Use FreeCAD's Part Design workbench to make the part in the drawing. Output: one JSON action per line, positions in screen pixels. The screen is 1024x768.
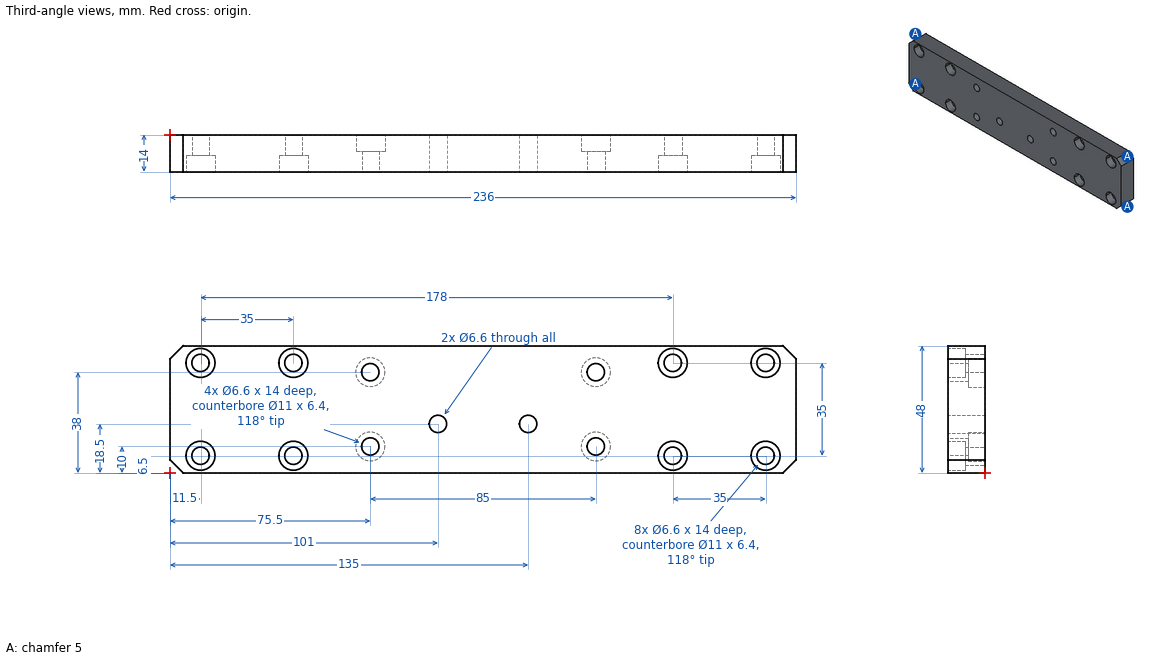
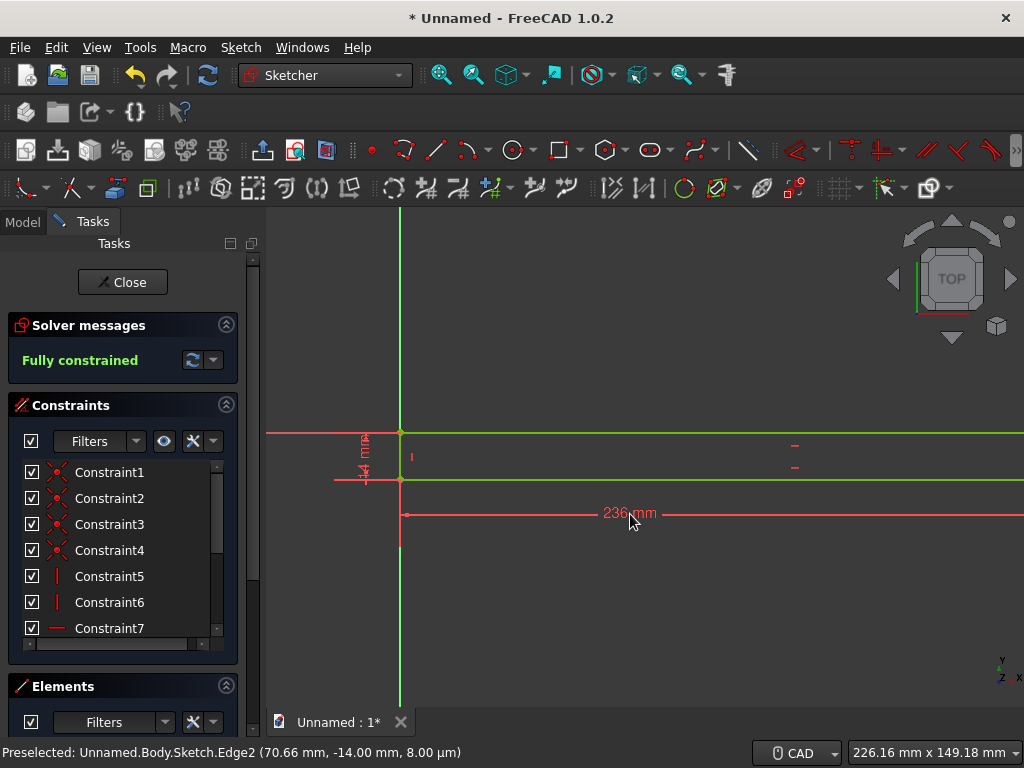
{"action": "left_click", "coordinate": [123, 282]}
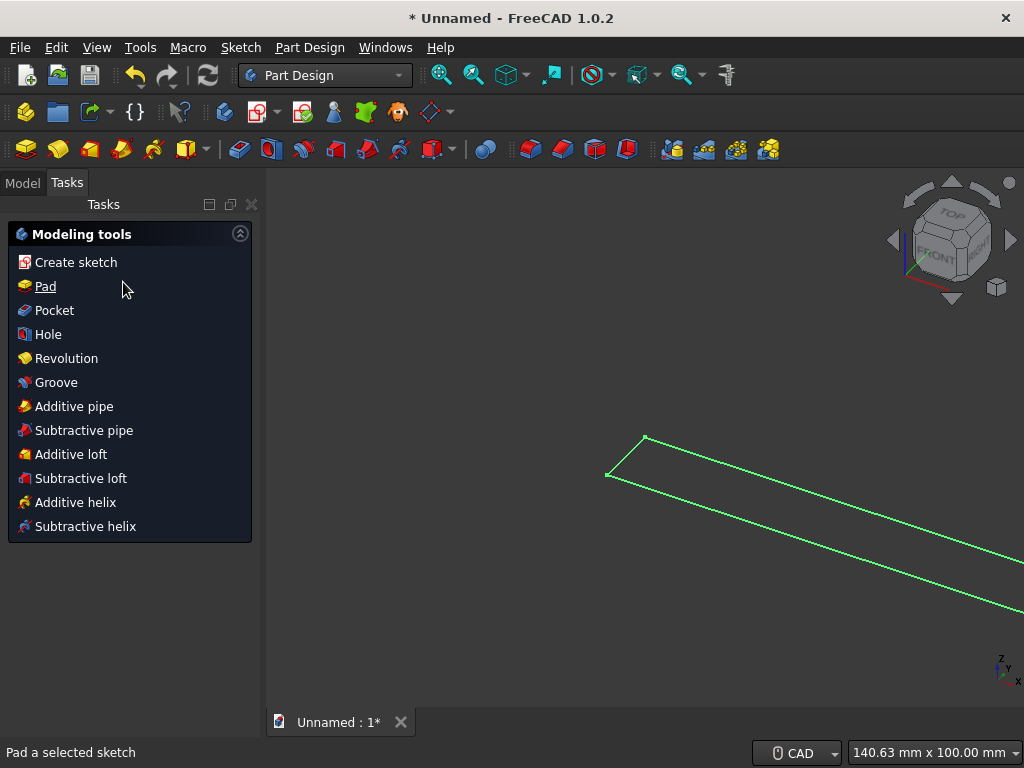
{"action": "left_click", "coordinate": [26, 150]}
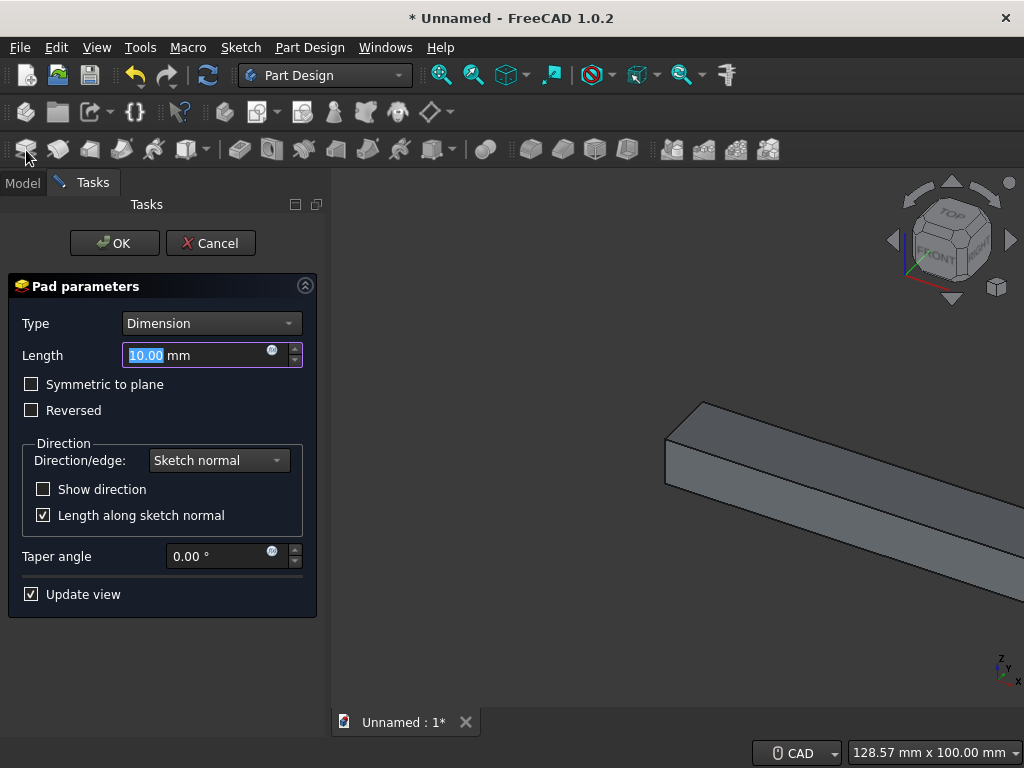
{"action": "type", "text": "48"}
{"action": "key", "text": "Tab"}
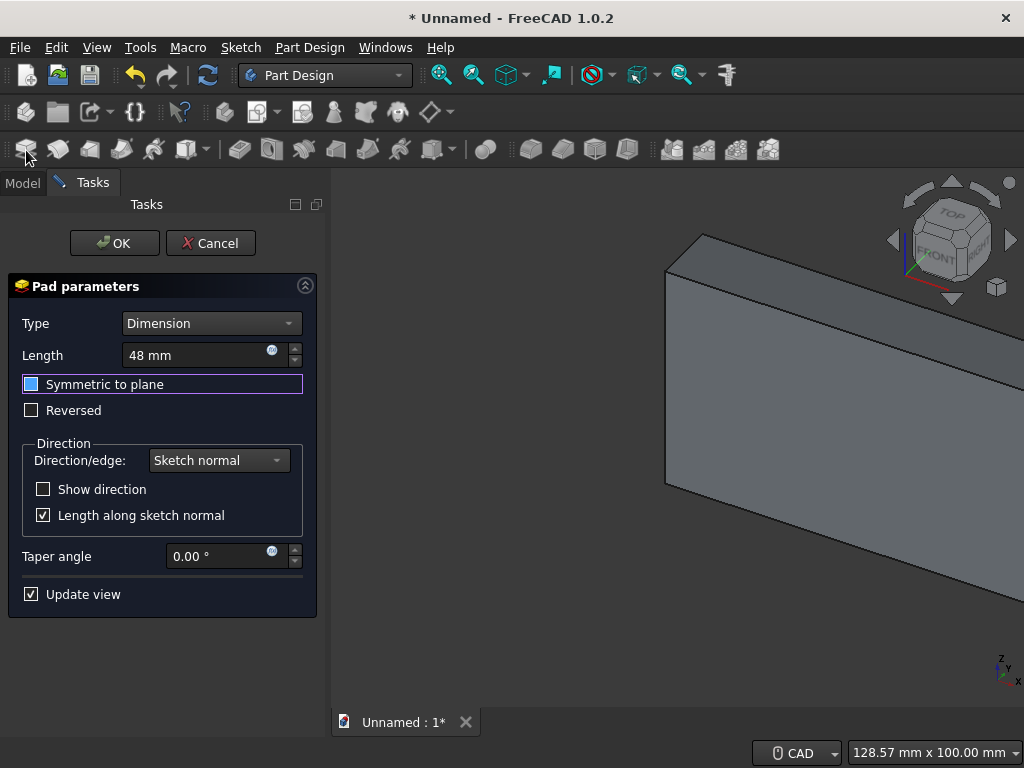
{"action": "left_click", "coordinate": [115, 243]}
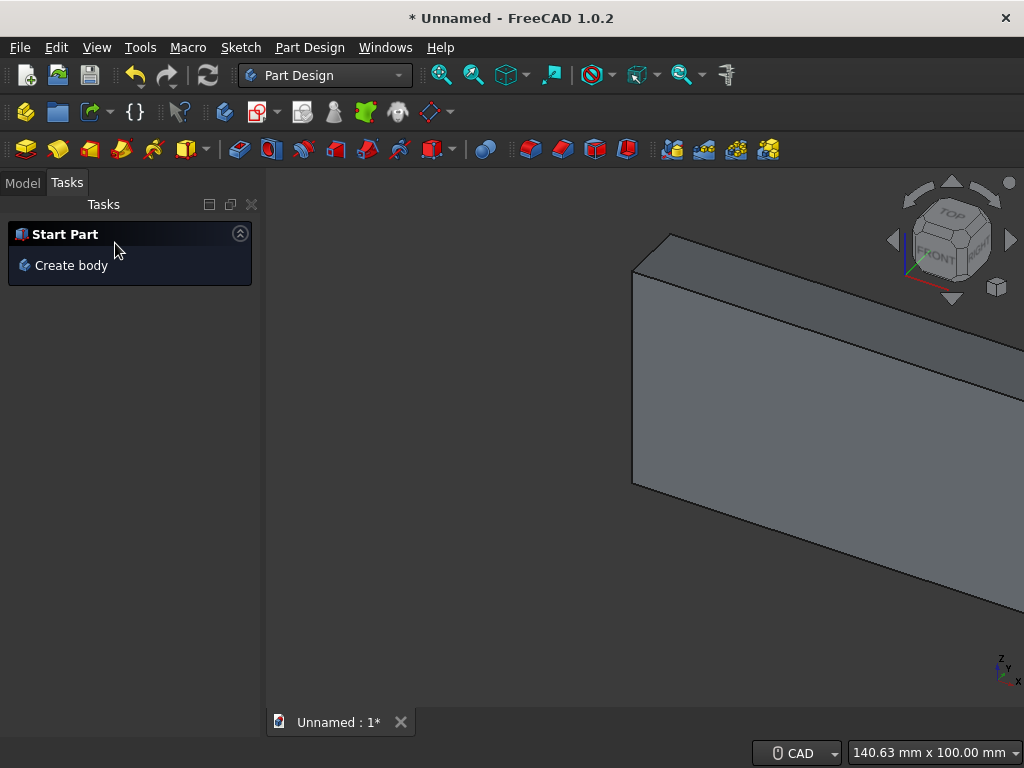
{"action": "left_click", "coordinate": [442, 76]}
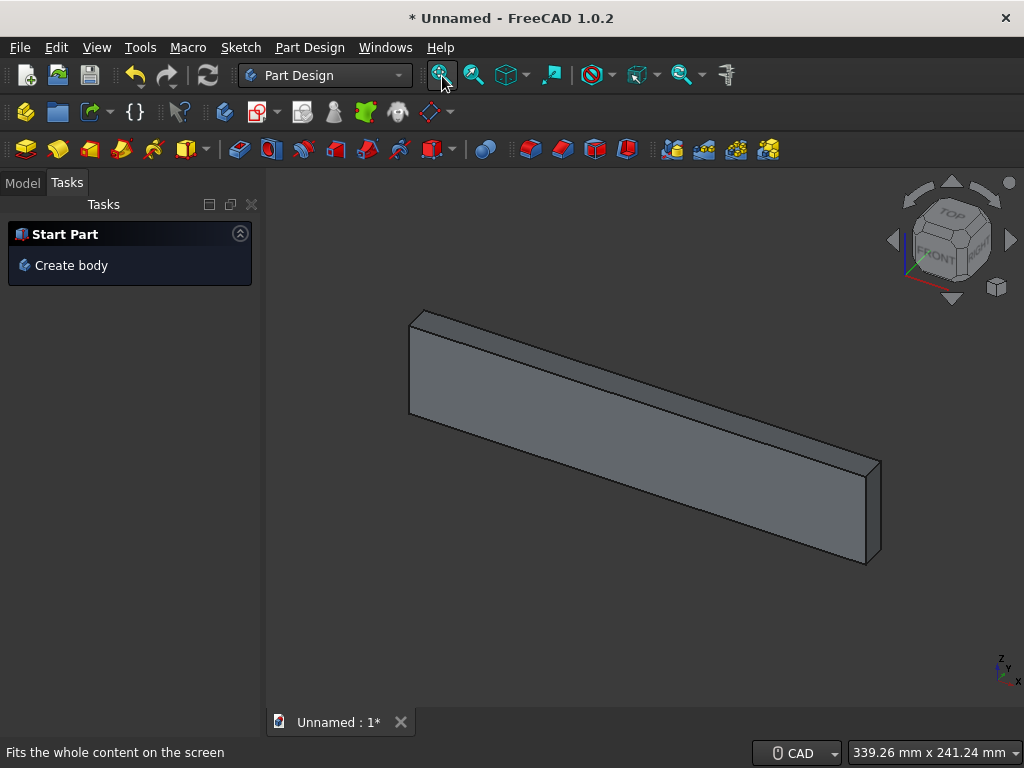
{"action": "left_click", "coordinate": [768, 487]}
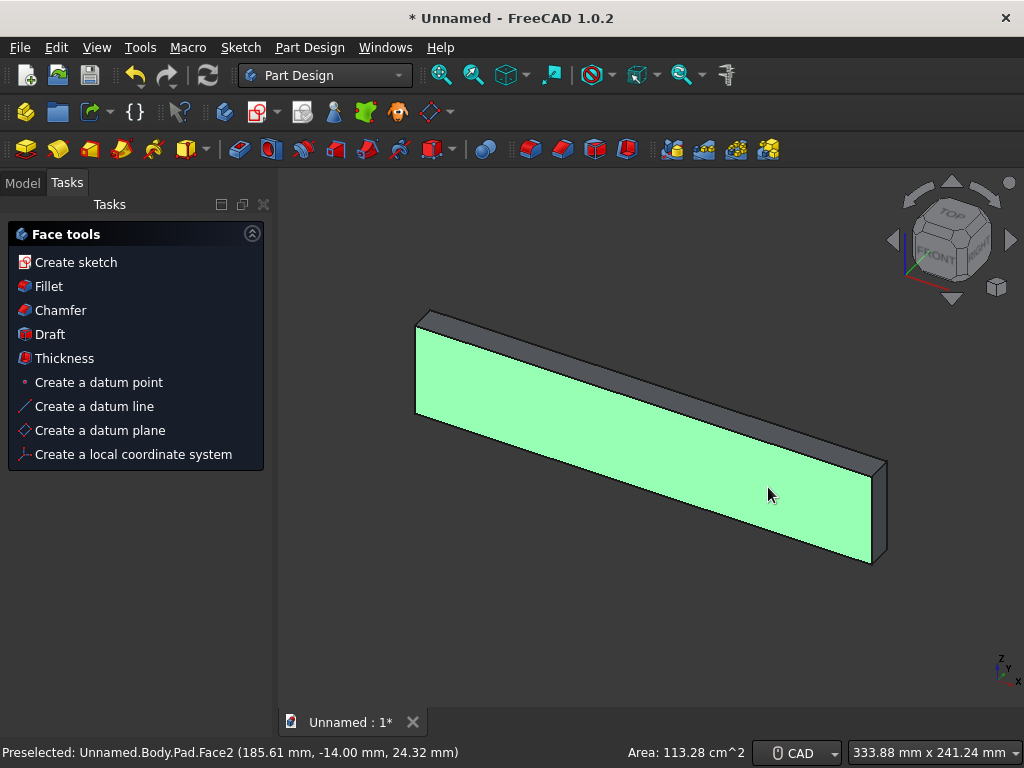
{"action": "left_click", "coordinate": [258, 112]}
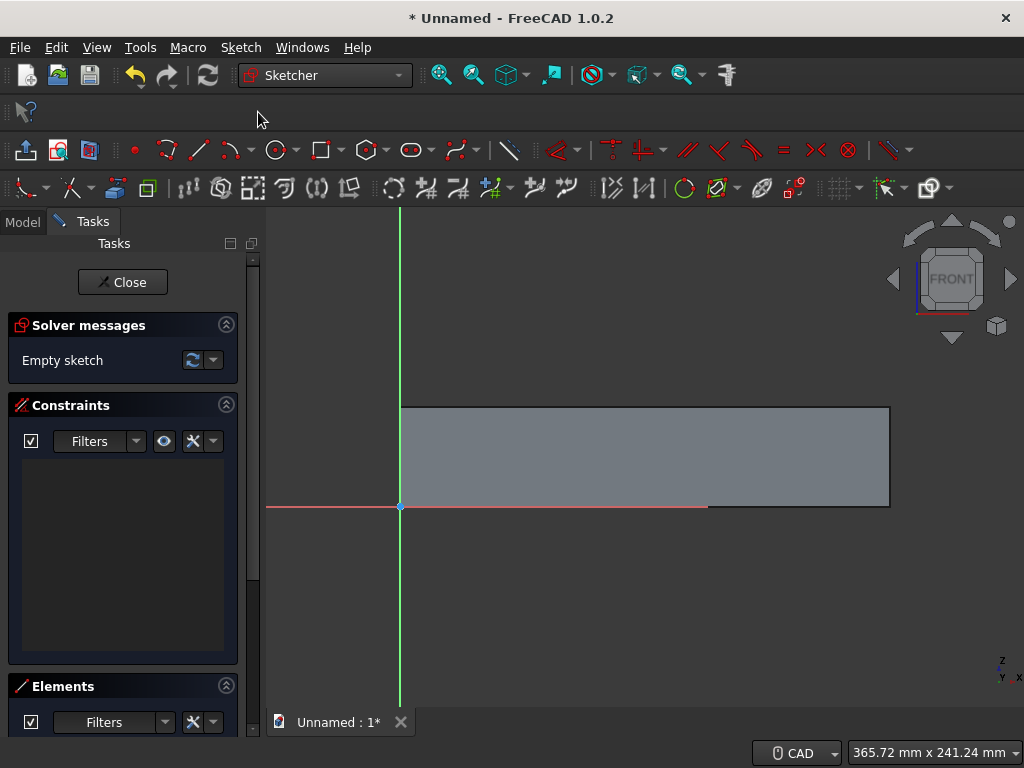
{"action": "scroll", "coordinate": [305, 442], "scroll_direction": "down", "scroll_amount": 1}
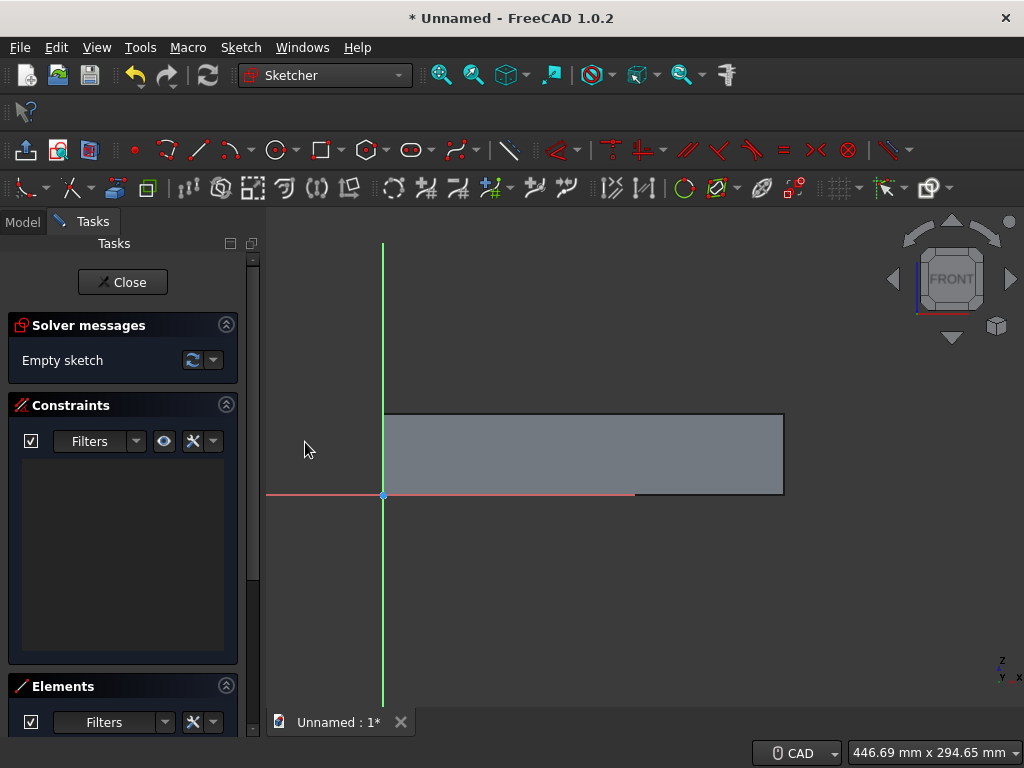
{"action": "left_click", "coordinate": [276, 150]}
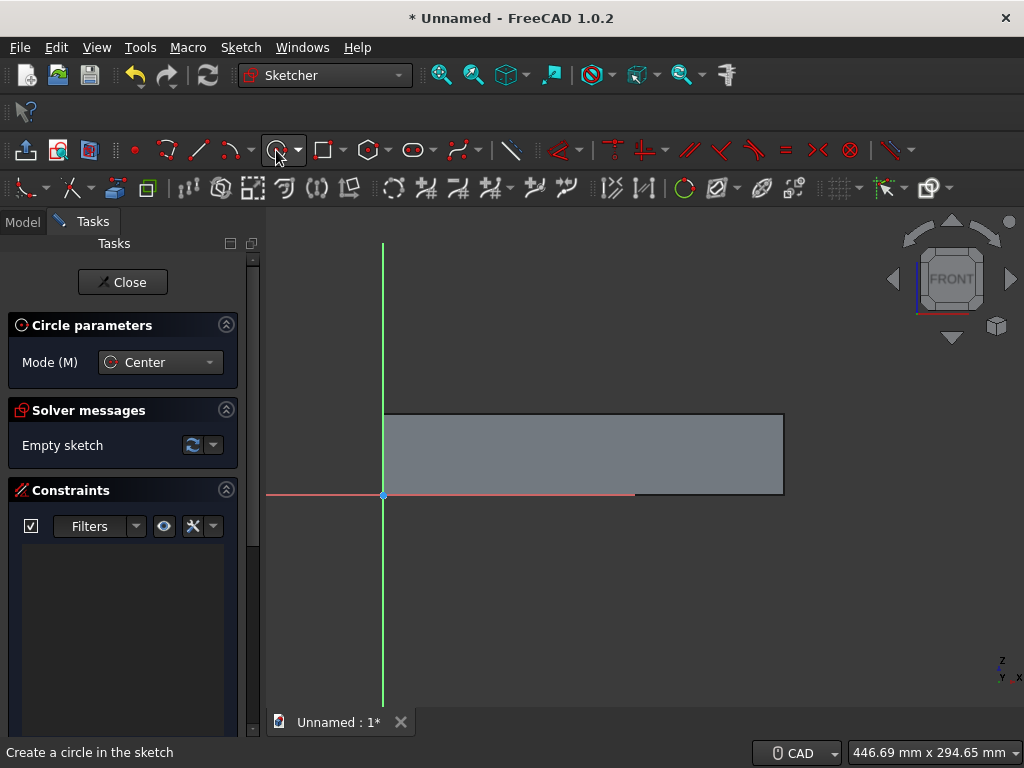
{"action": "scroll", "coordinate": [764, 484], "scroll_direction": "up", "scroll_amount": 7}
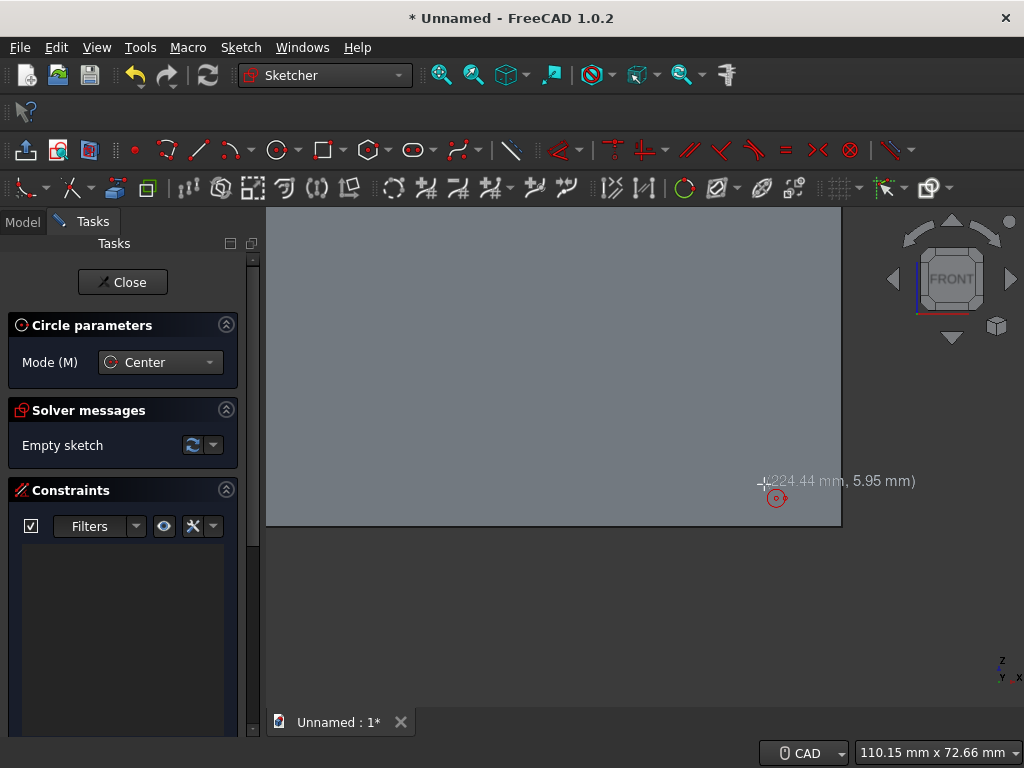
{"action": "left_click", "coordinate": [762, 483]}
{"action": "left_click", "coordinate": [778, 467]}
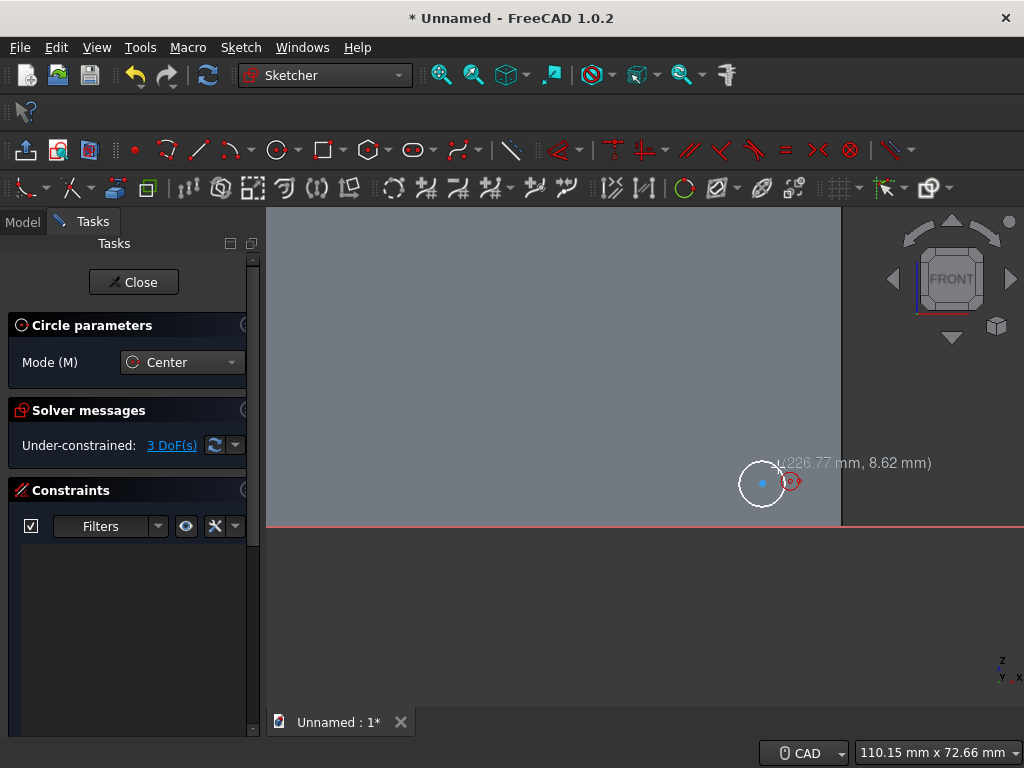
{"action": "left_click", "coordinate": [522, 483]}
{"action": "left_click", "coordinate": [538, 467]}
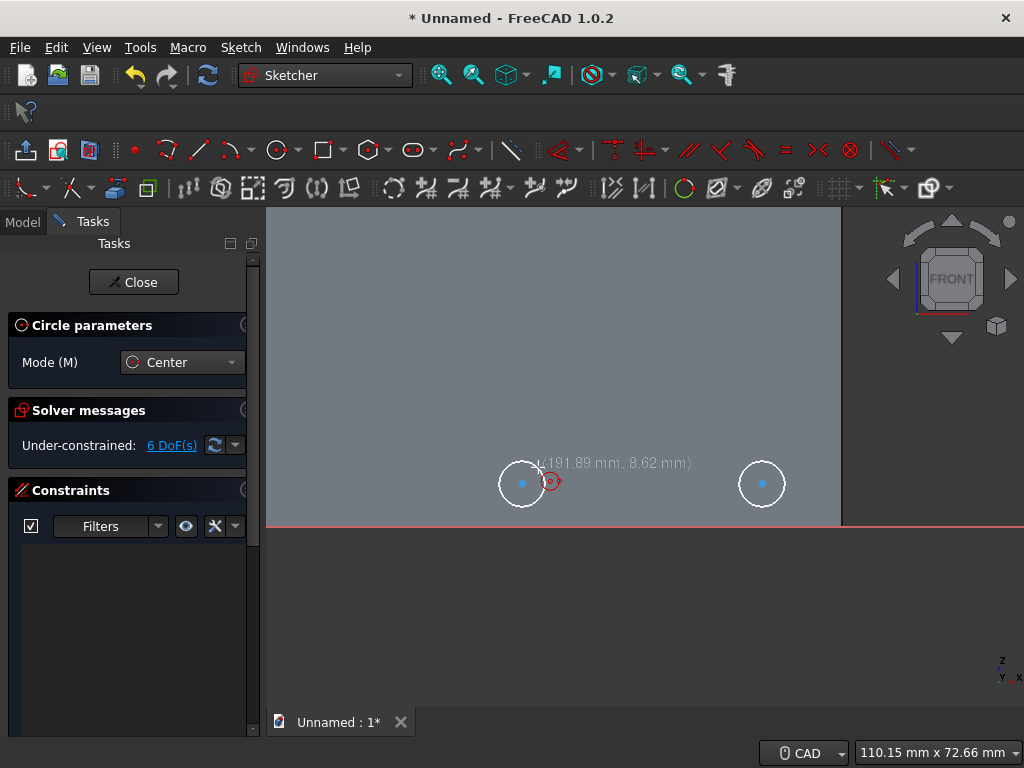
{"action": "scroll", "coordinate": [765, 484], "scroll_direction": "down", "scroll_amount": 7}